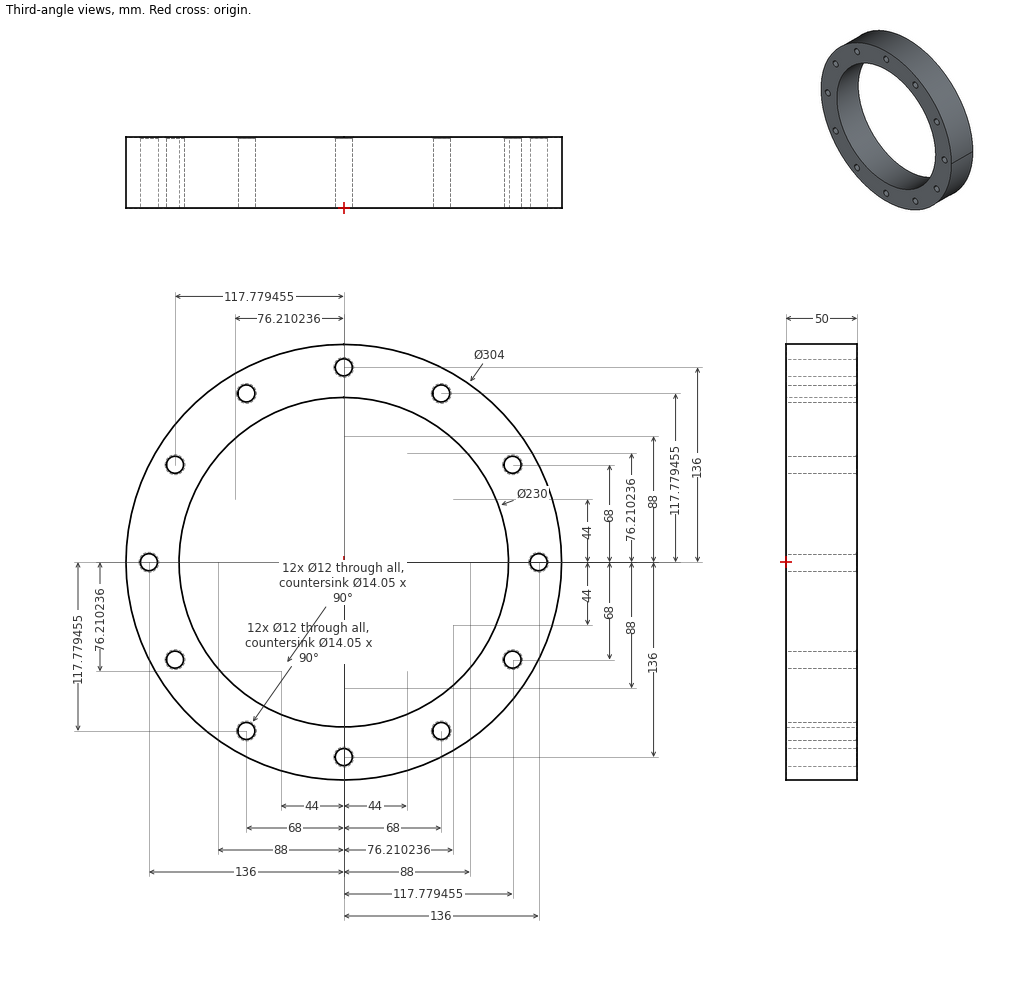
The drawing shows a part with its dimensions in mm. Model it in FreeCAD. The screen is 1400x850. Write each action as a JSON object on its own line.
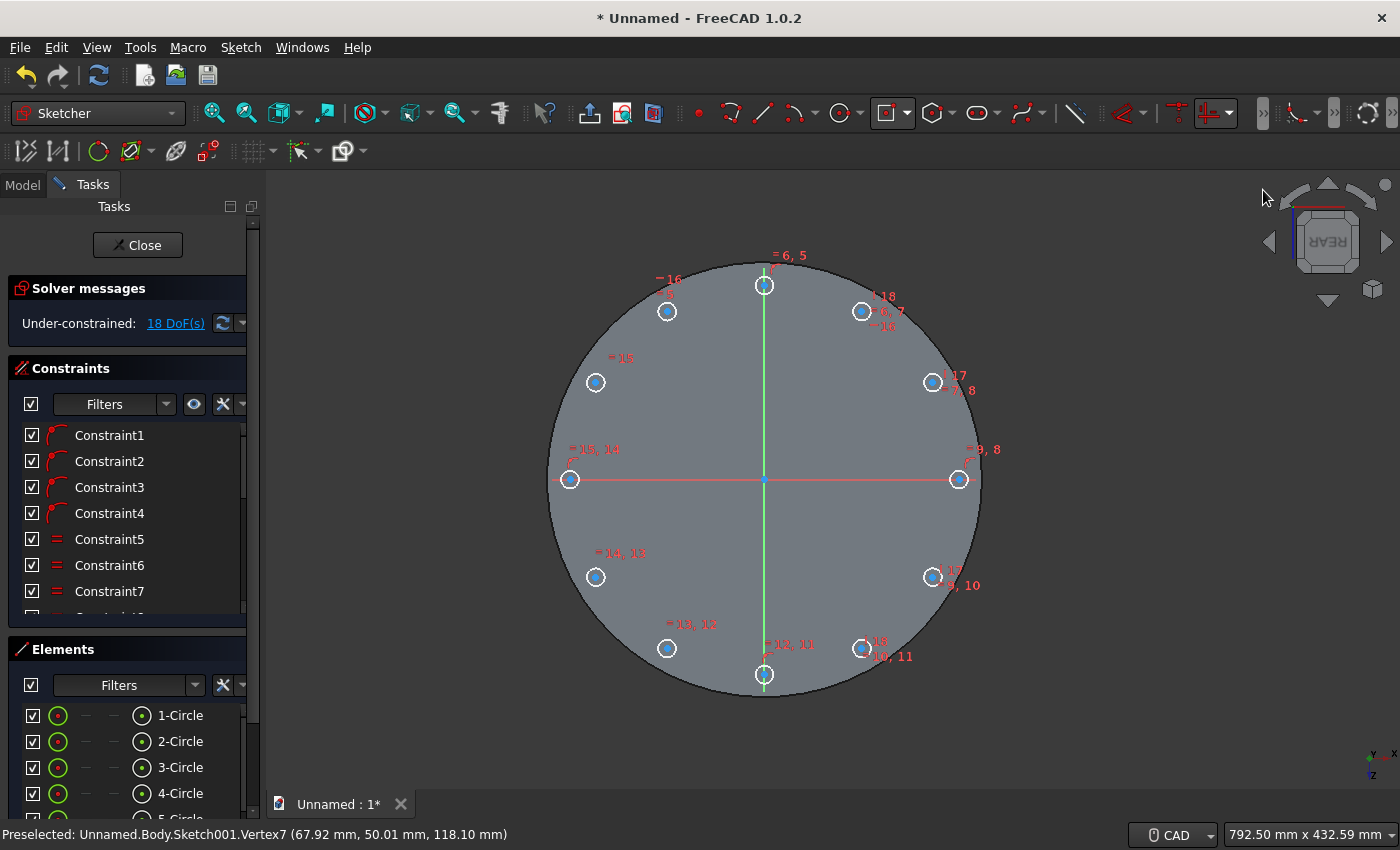
{"action": "left_click", "coordinate": [667, 312]}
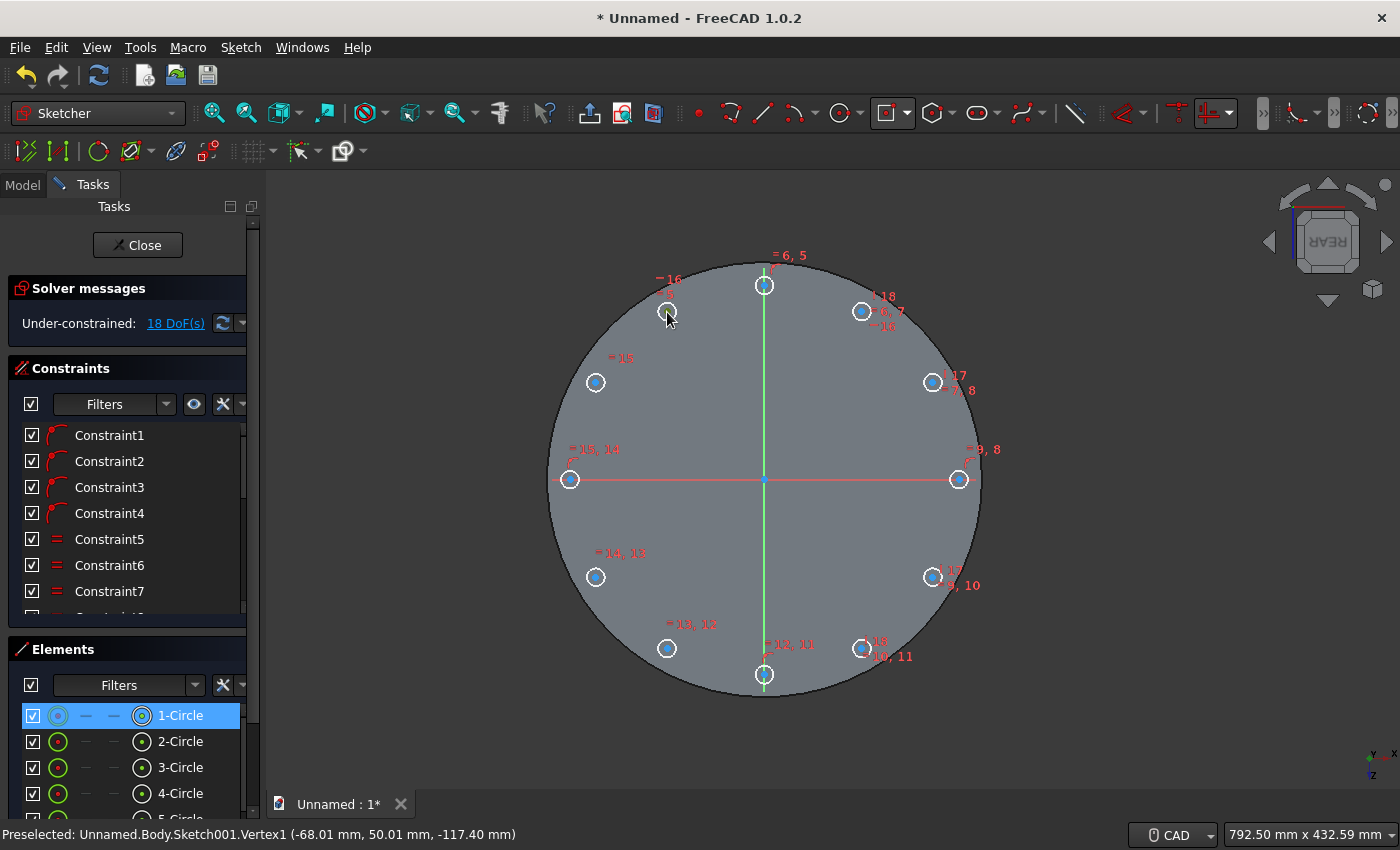
{"action": "left_click", "coordinate": [667, 649]}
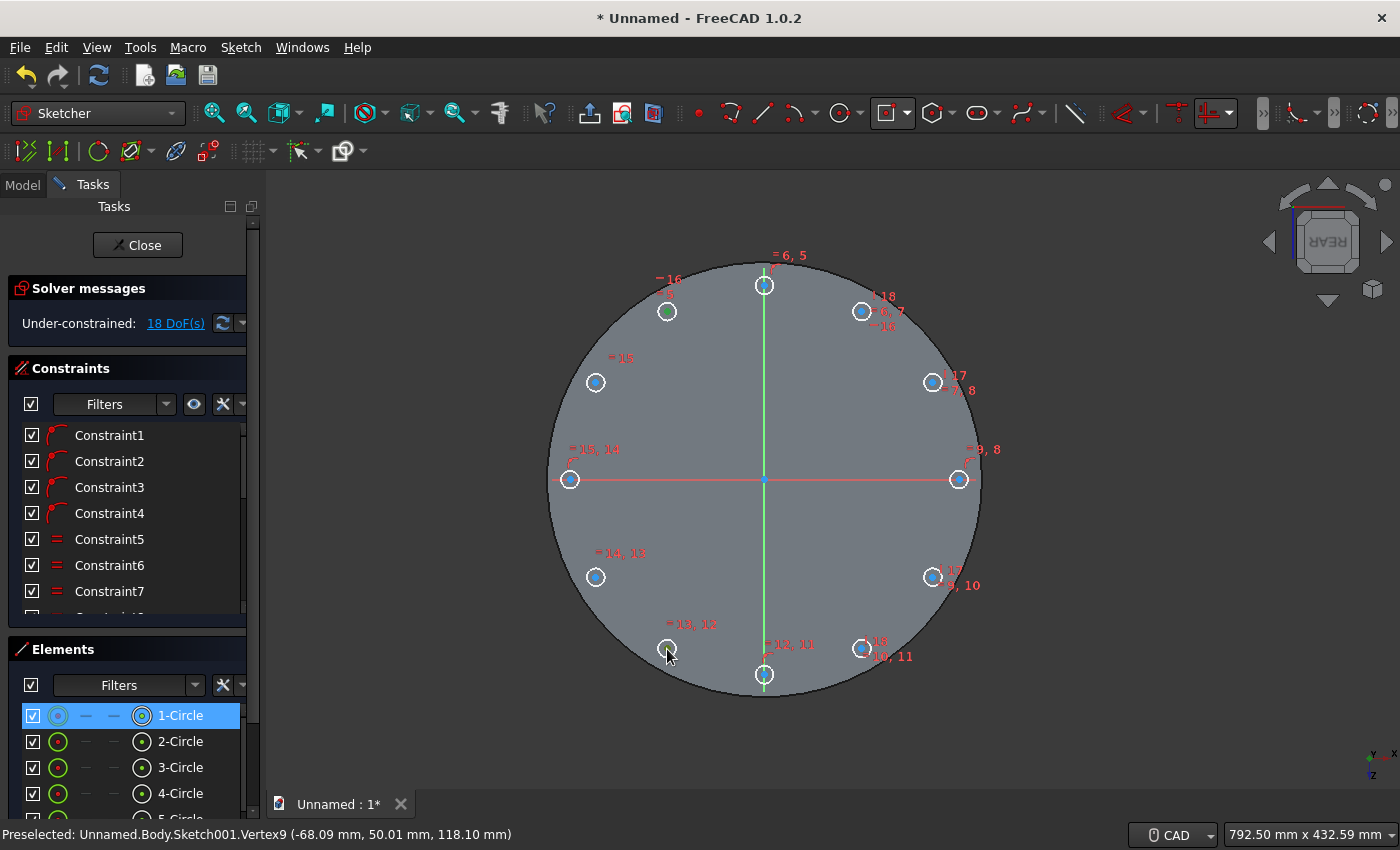
{"action": "left_click", "coordinate": [1232, 114]}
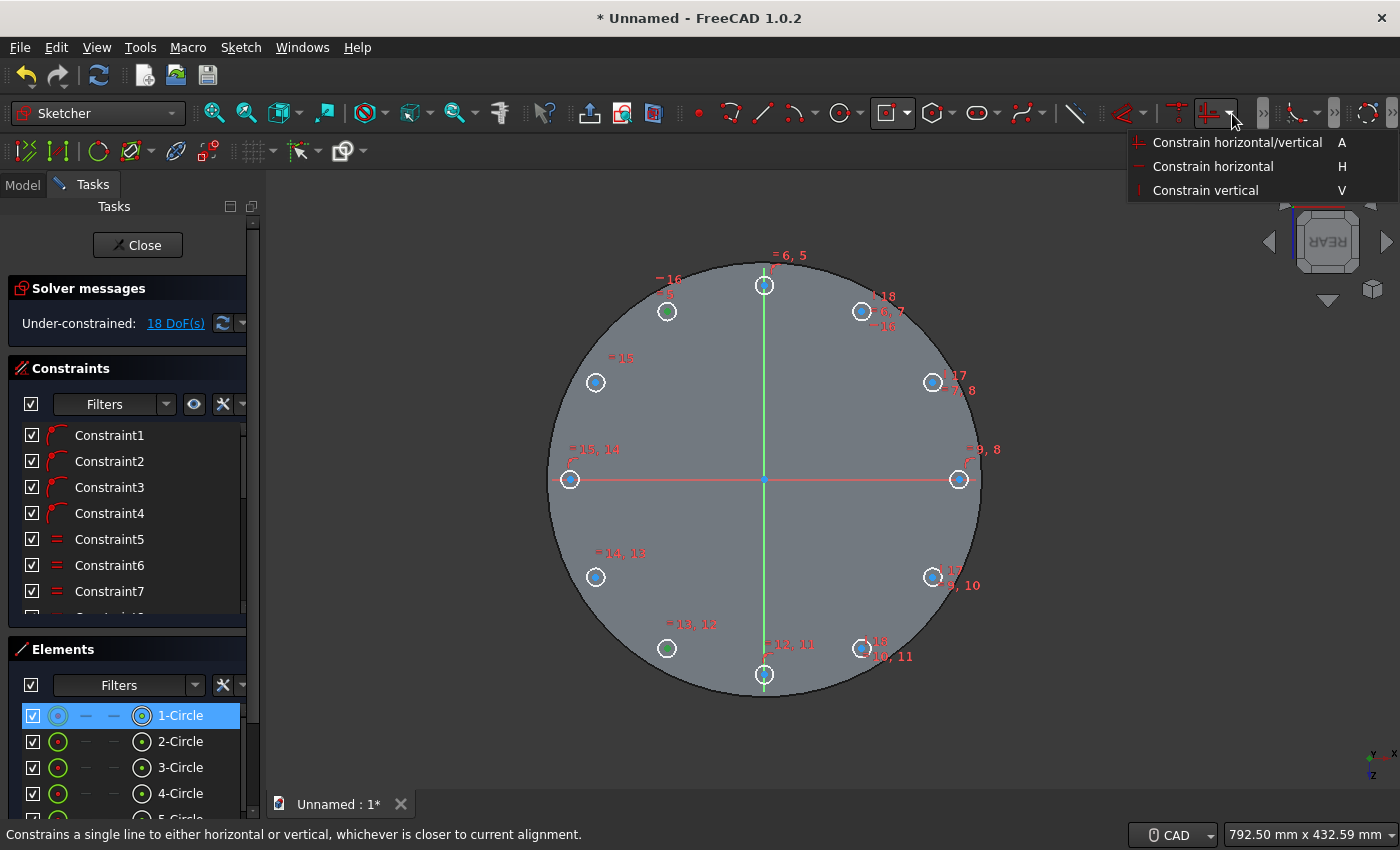
{"action": "left_click", "coordinate": [1263, 190]}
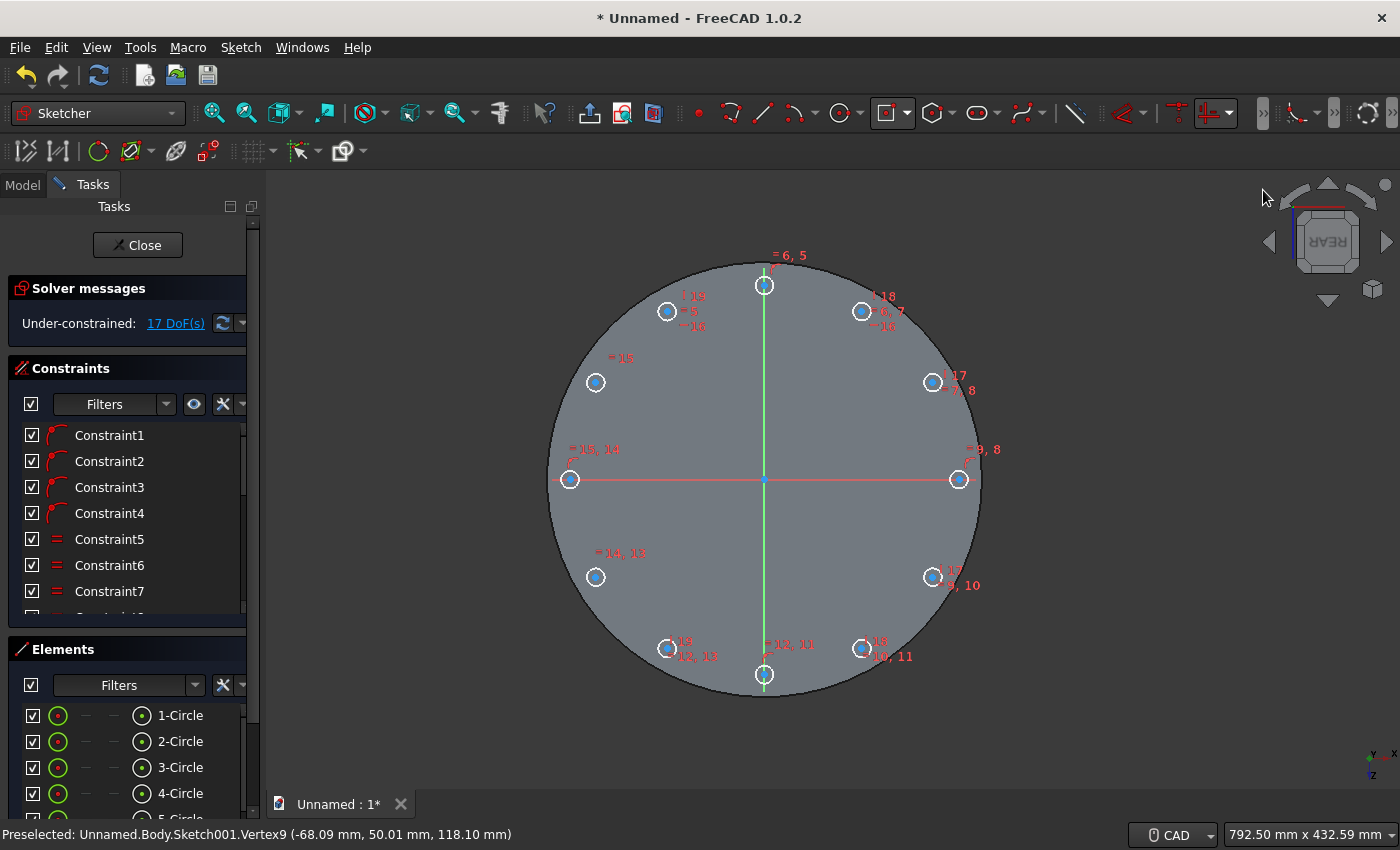
{"action": "left_click", "coordinate": [860, 651]}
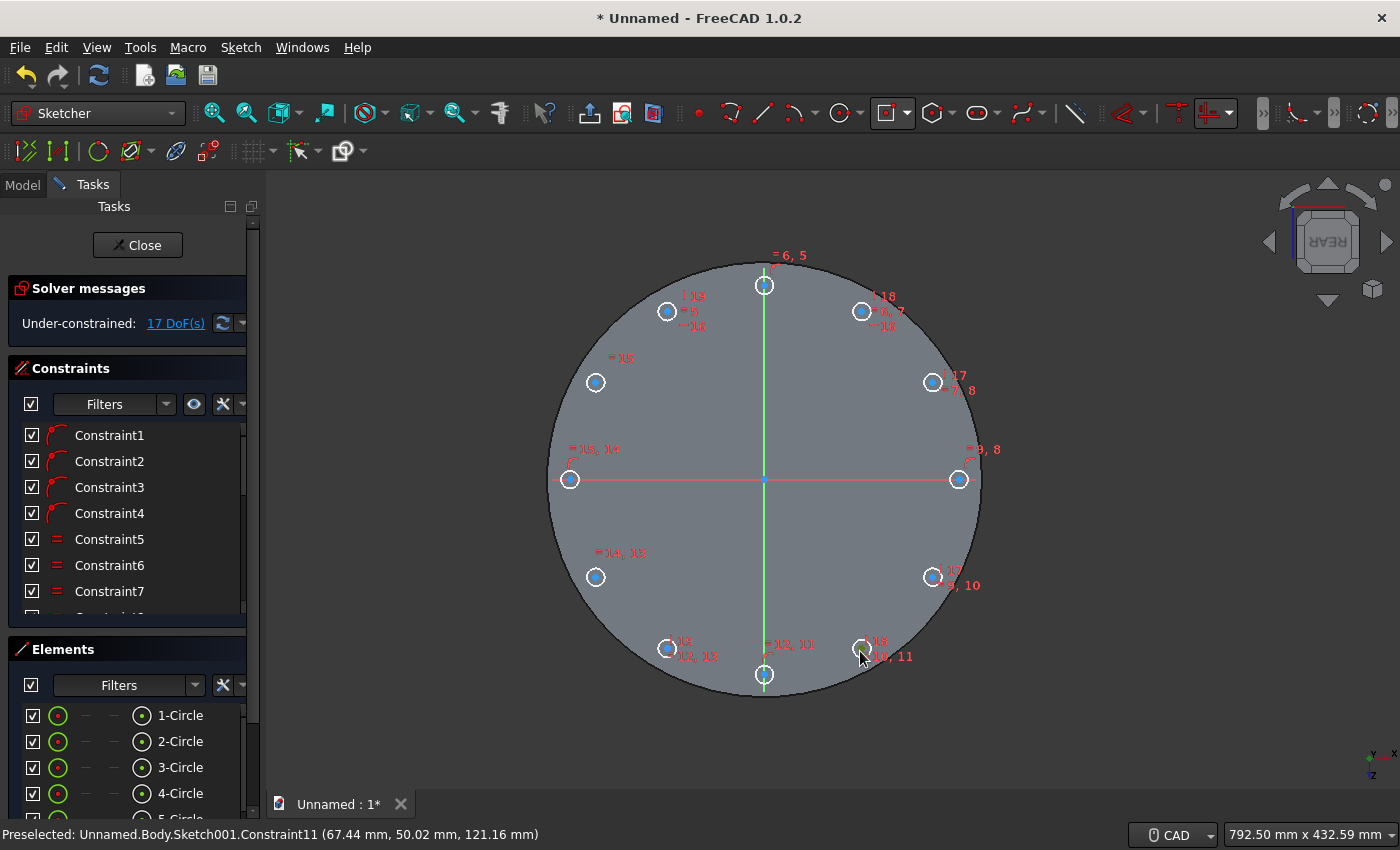
{"action": "left_click", "coordinate": [665, 651]}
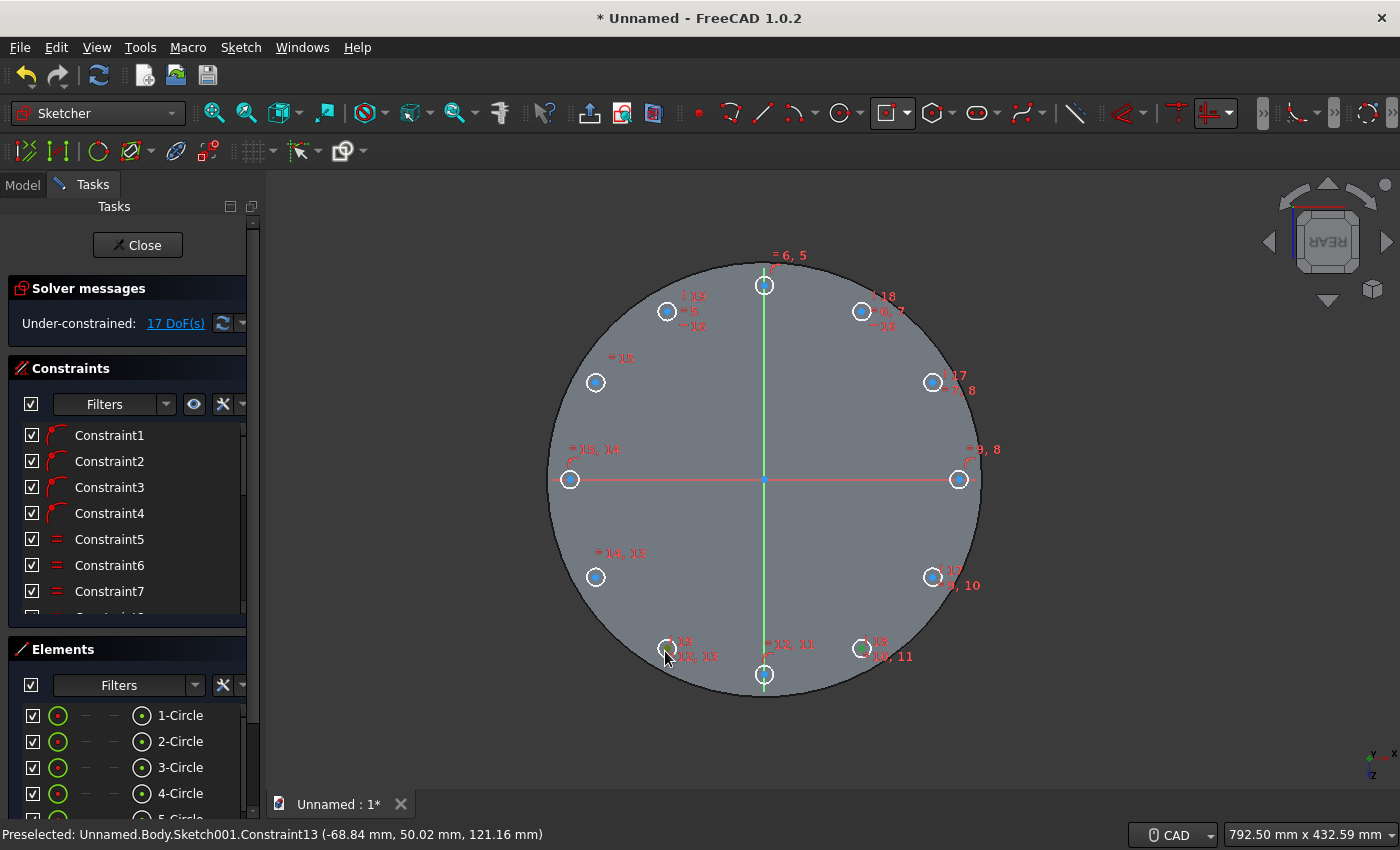
{"action": "key", "text": "h"}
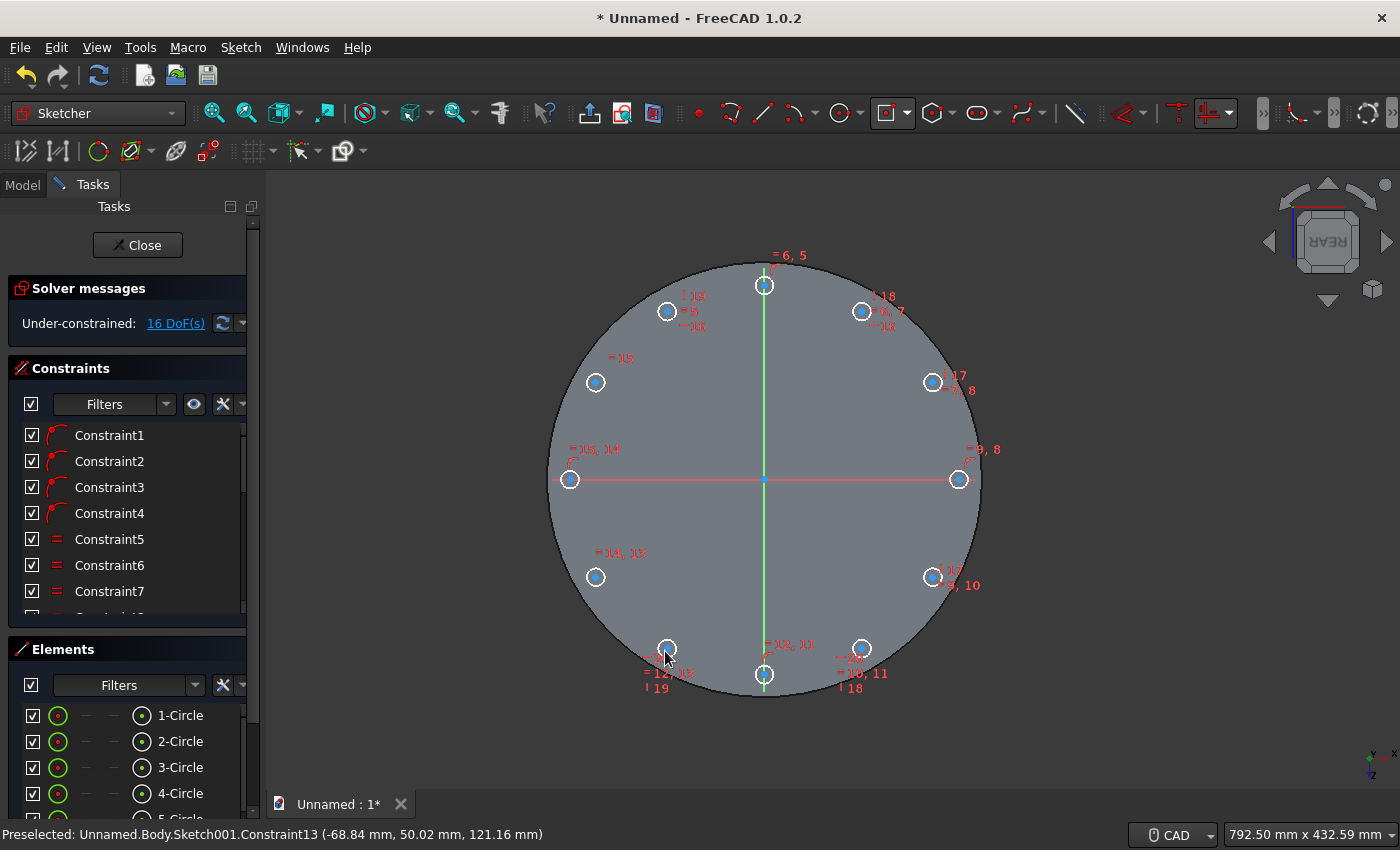
{"action": "left_click", "coordinate": [933, 577]}